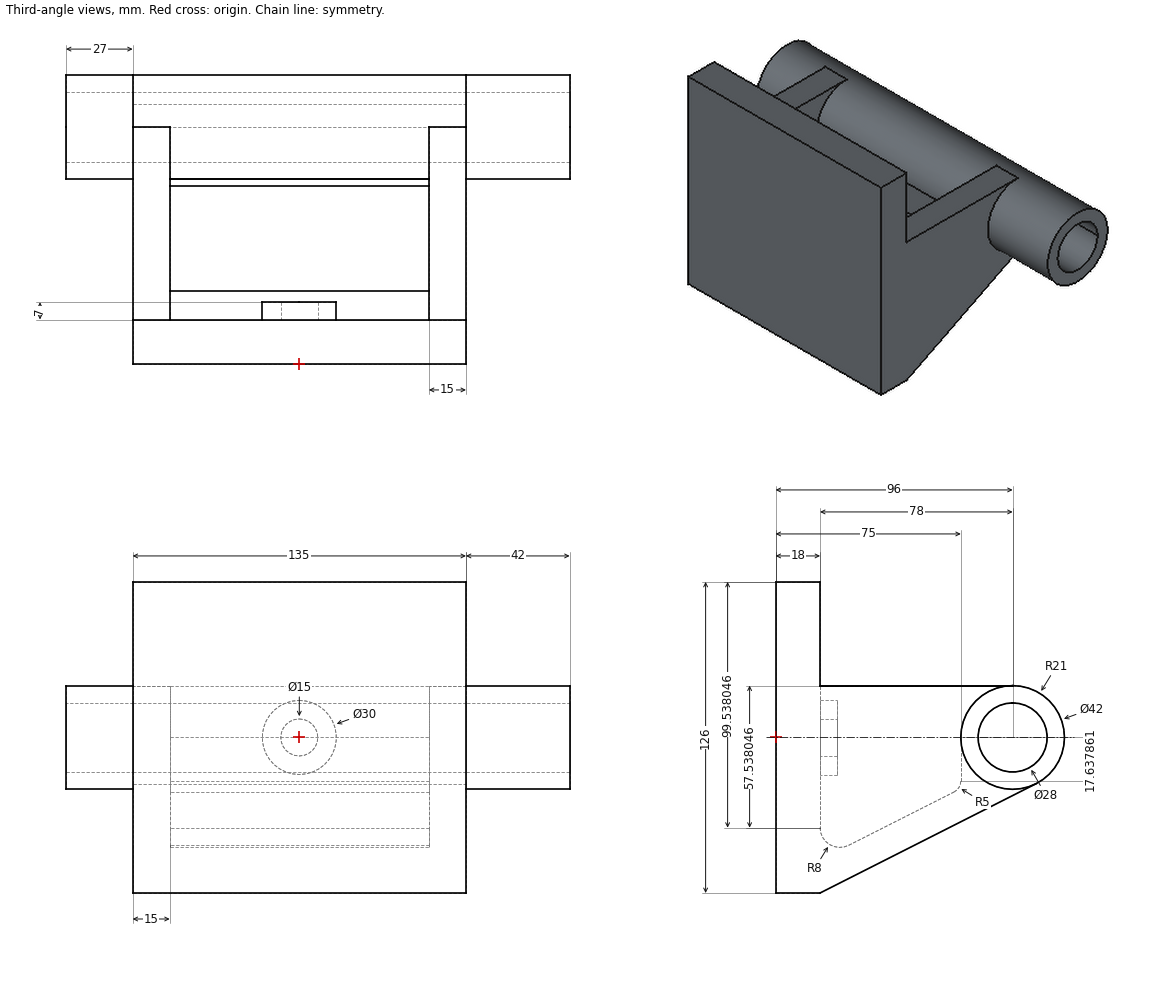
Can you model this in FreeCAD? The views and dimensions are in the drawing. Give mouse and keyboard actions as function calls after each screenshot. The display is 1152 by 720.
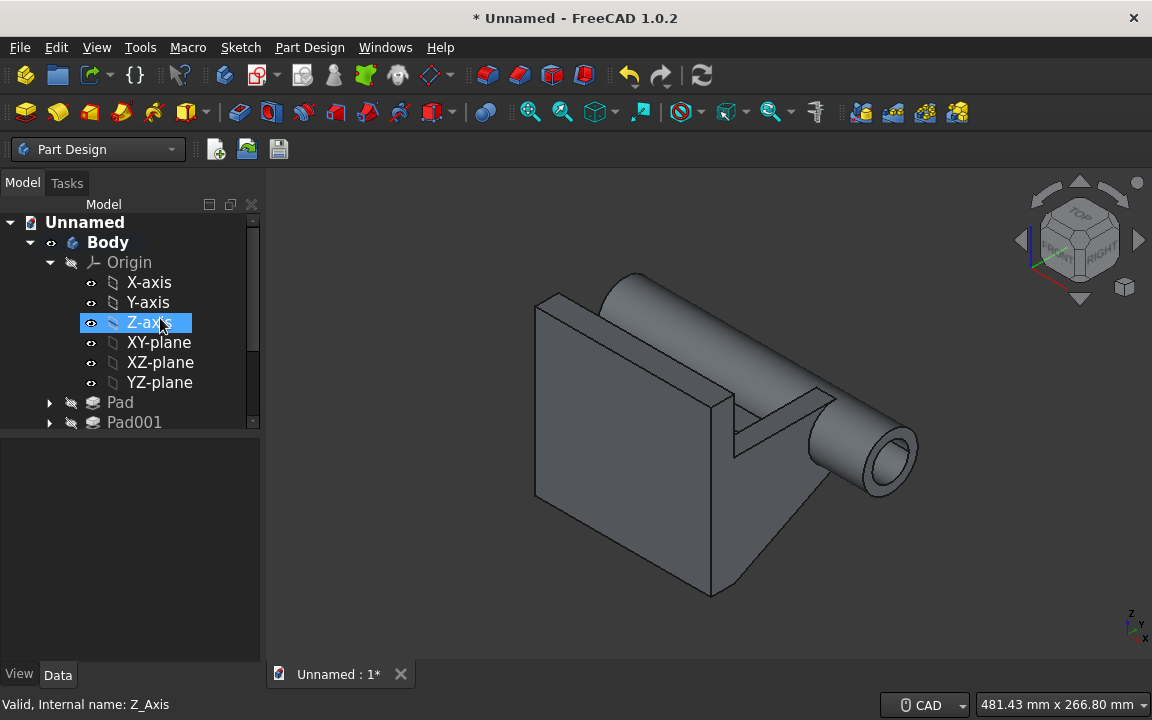
click(136, 383)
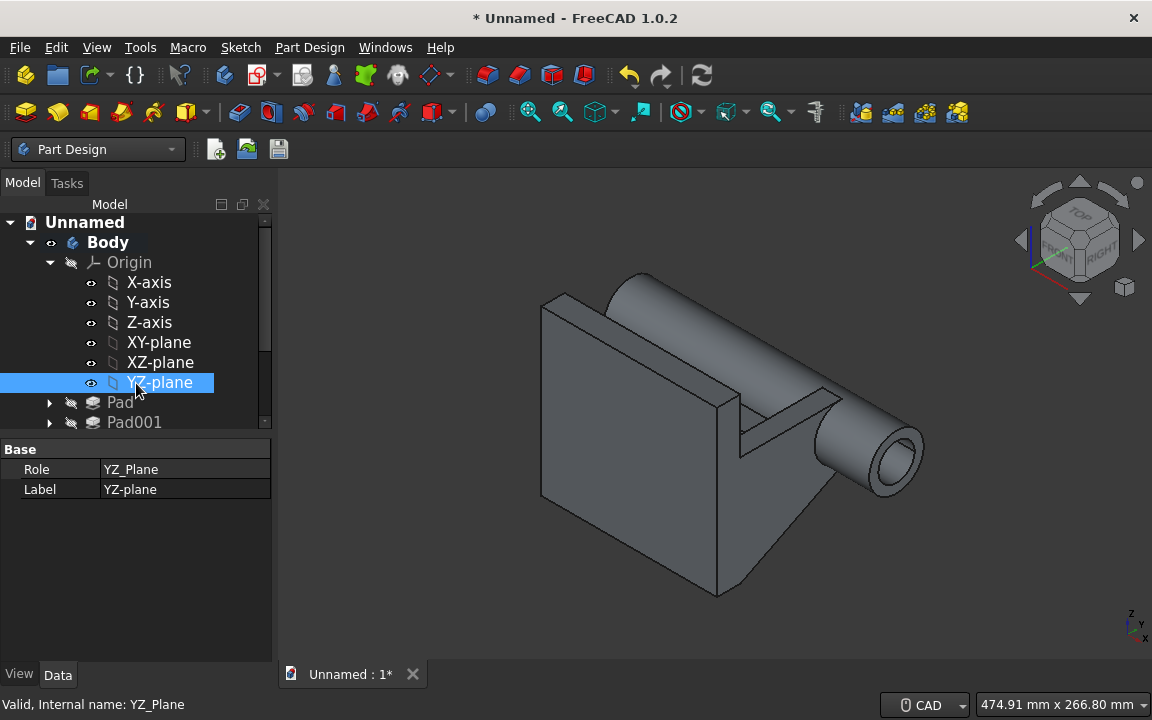
click(430, 76)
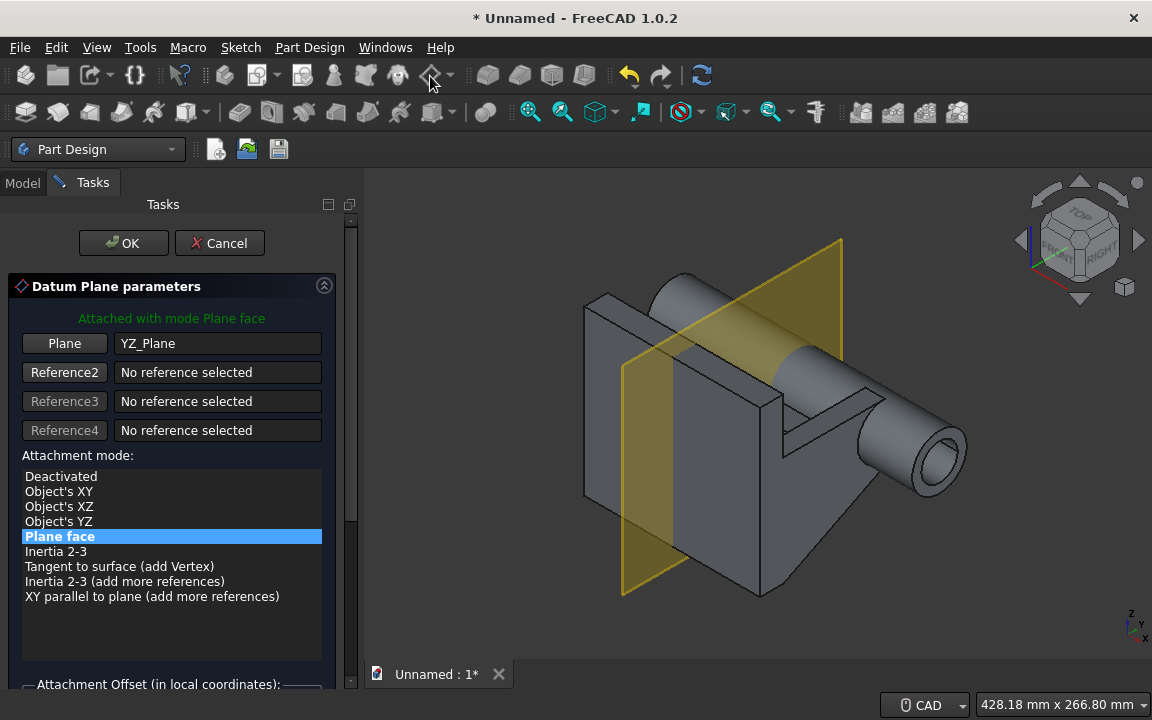
scroll(351, 451, down, 3)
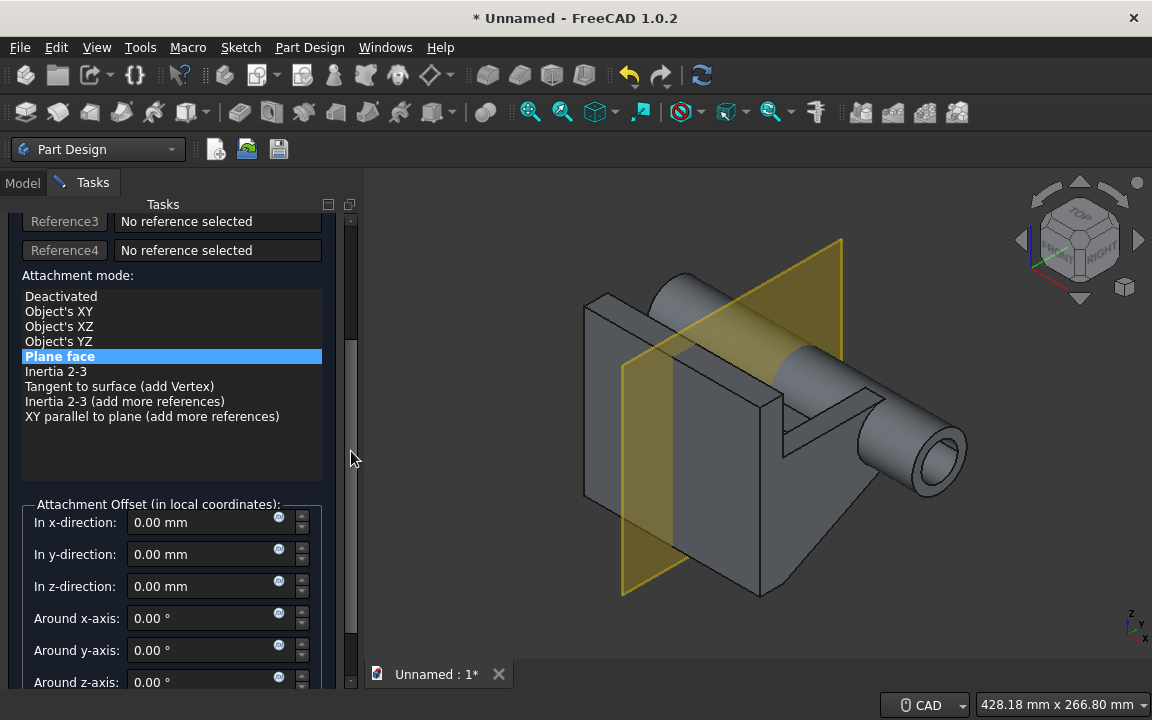
triple_click(210, 586)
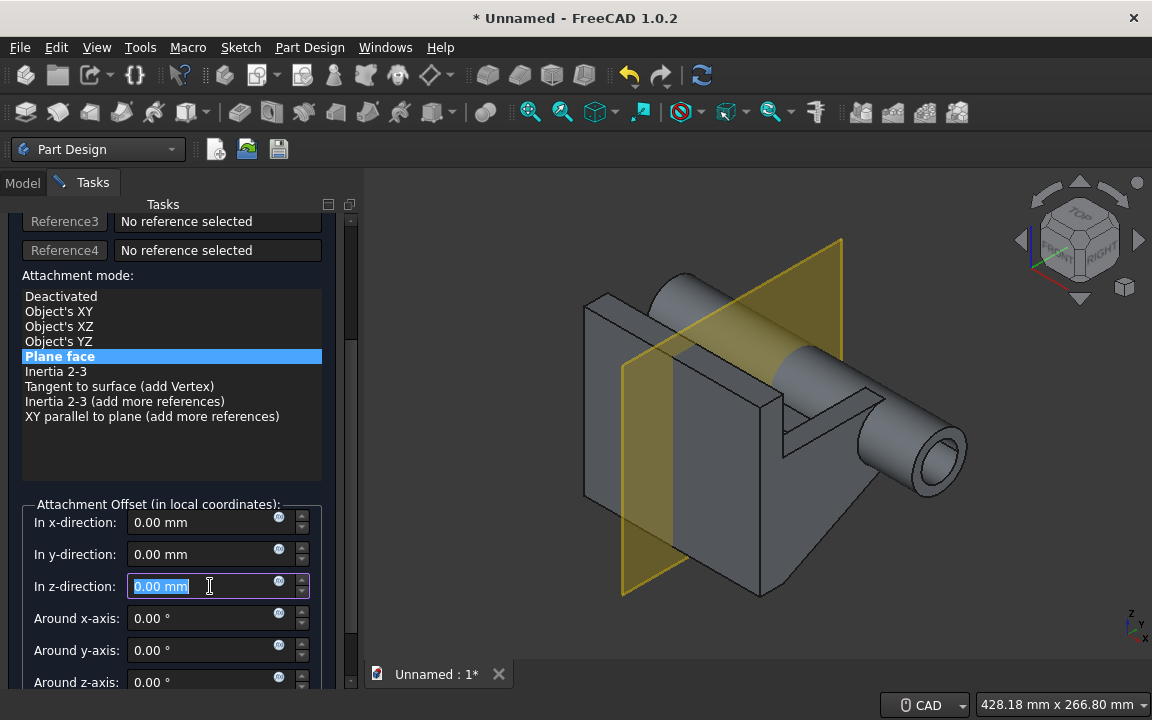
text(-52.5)
key(Tab)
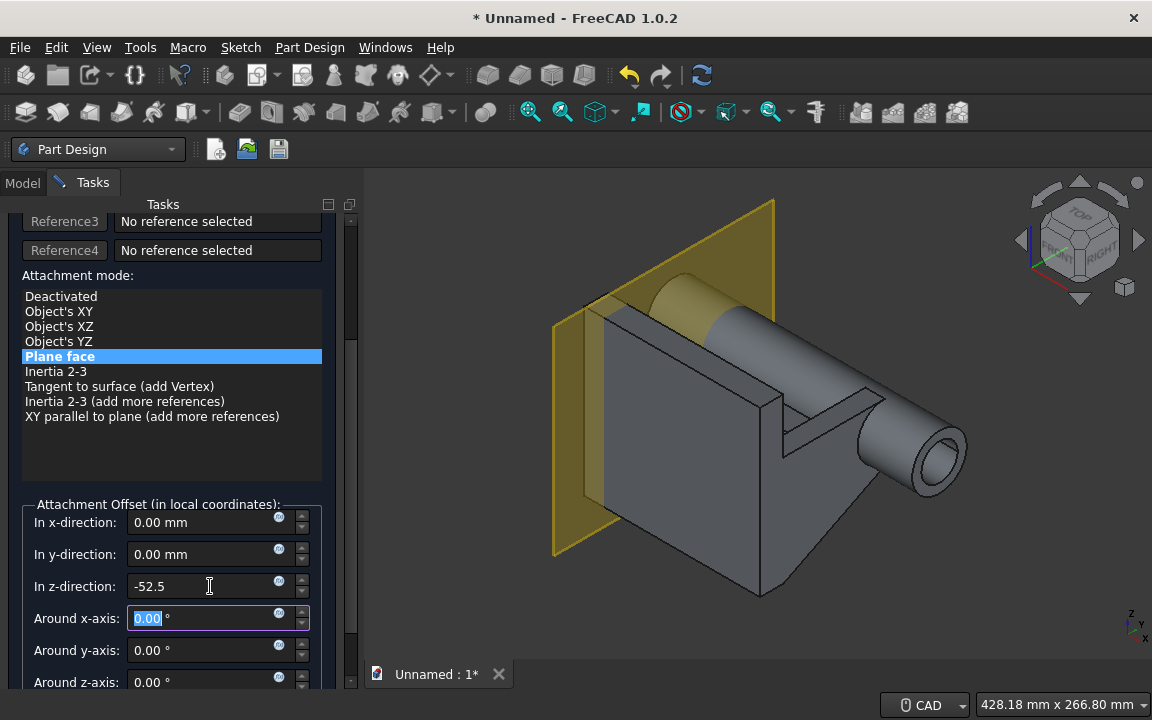
scroll(351, 451, up, 4)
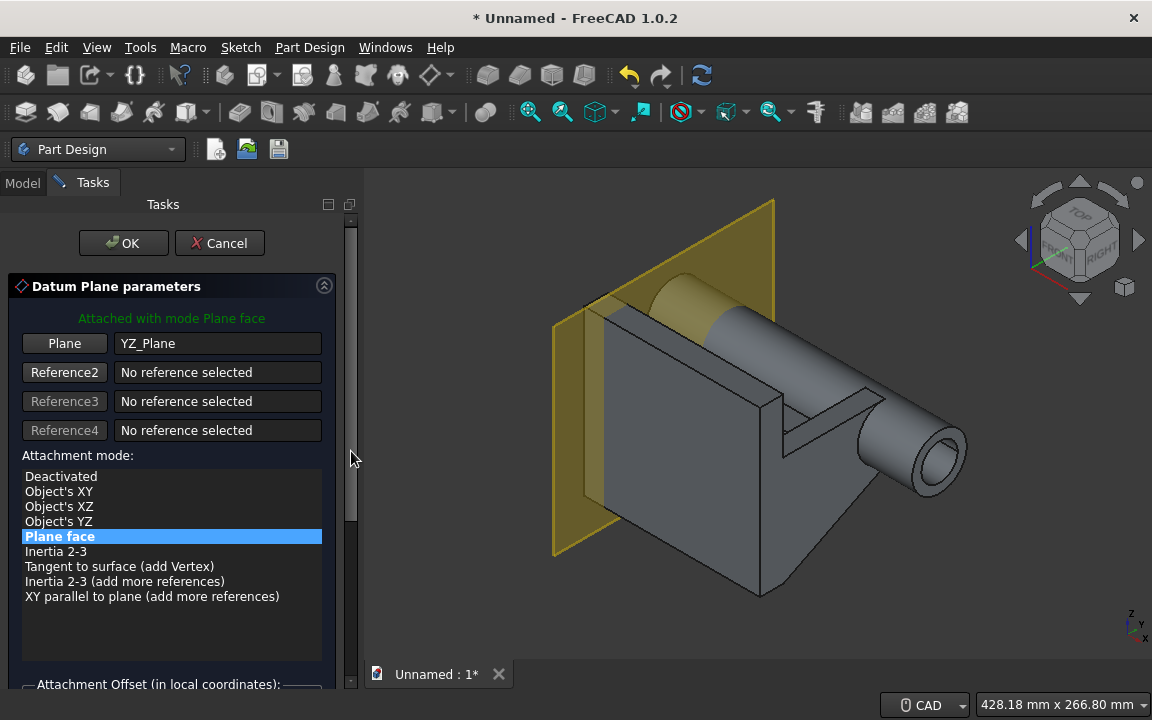
click(124, 243)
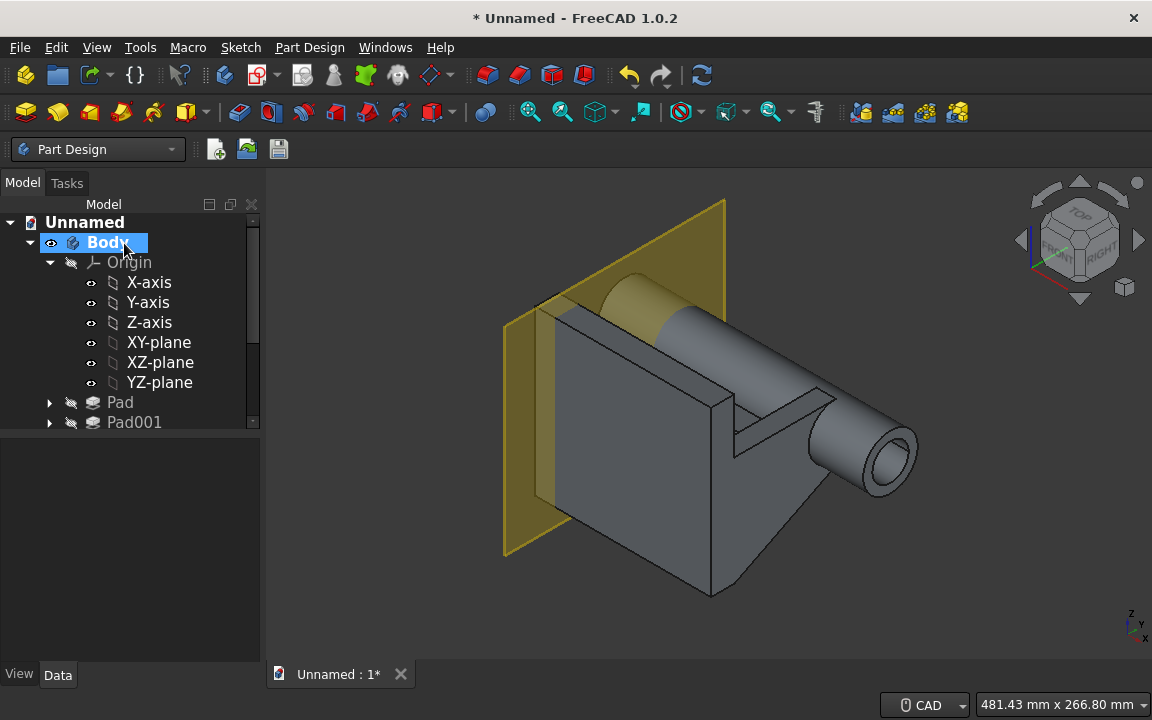
scroll(100, 318, down, 3)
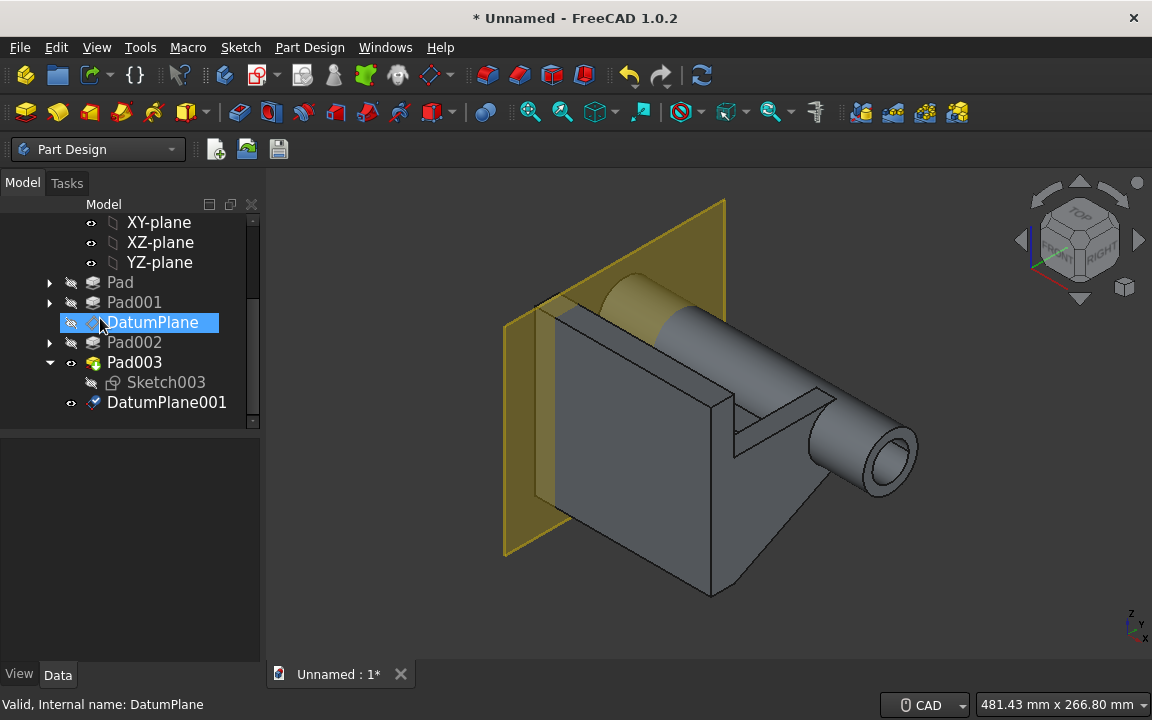
click(116, 403)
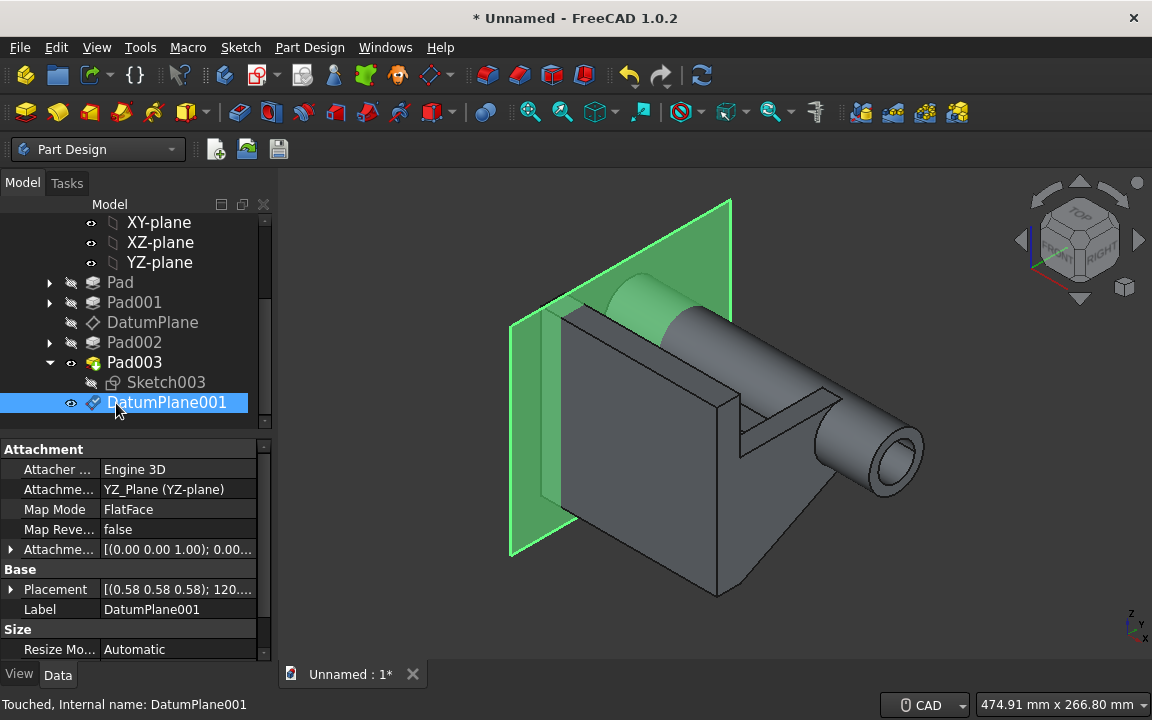
click(258, 76)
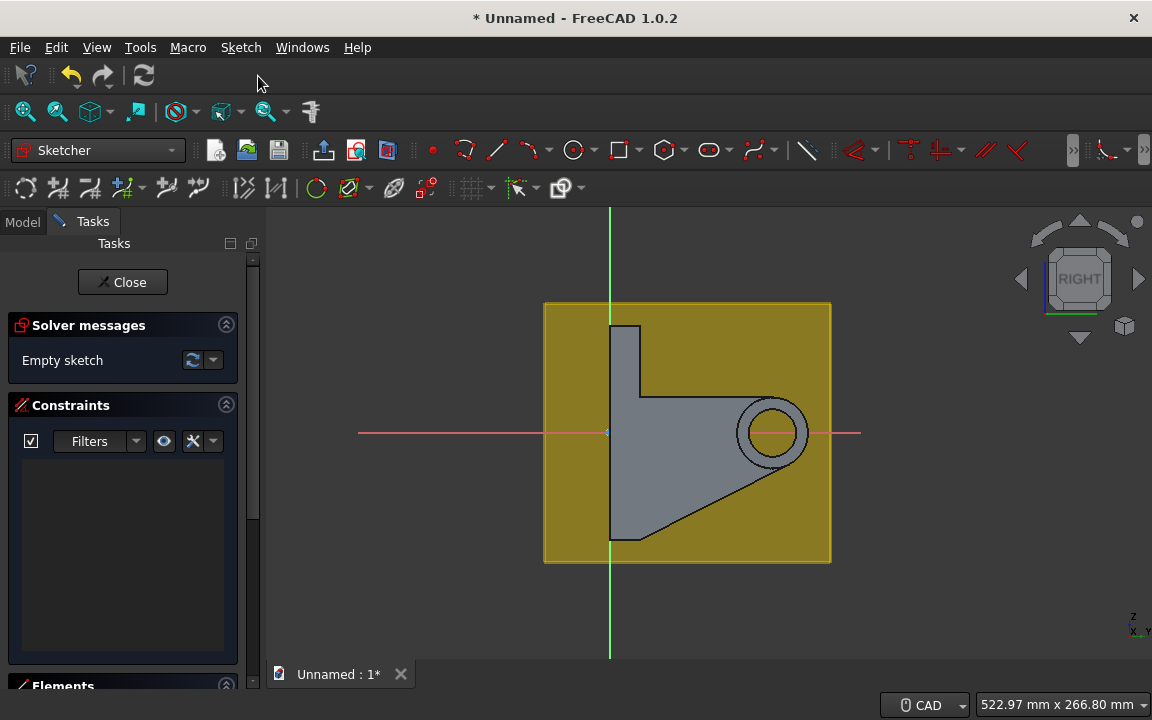
click(388, 150)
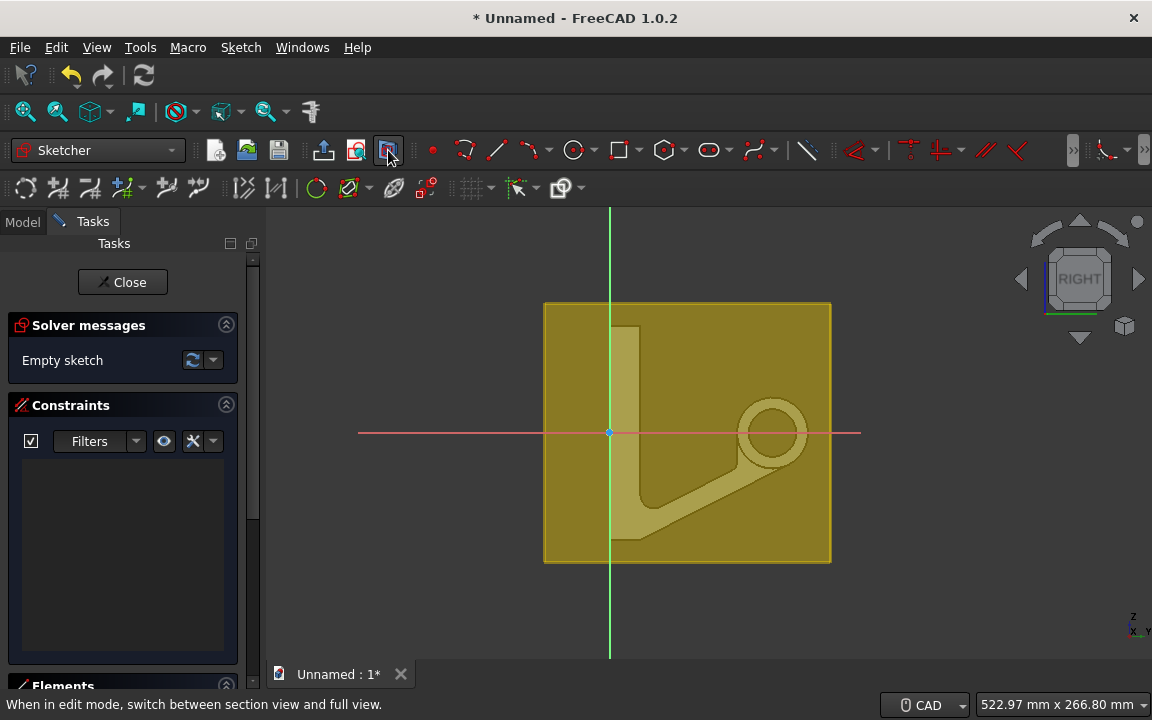
scroll(721, 463, up, 5)